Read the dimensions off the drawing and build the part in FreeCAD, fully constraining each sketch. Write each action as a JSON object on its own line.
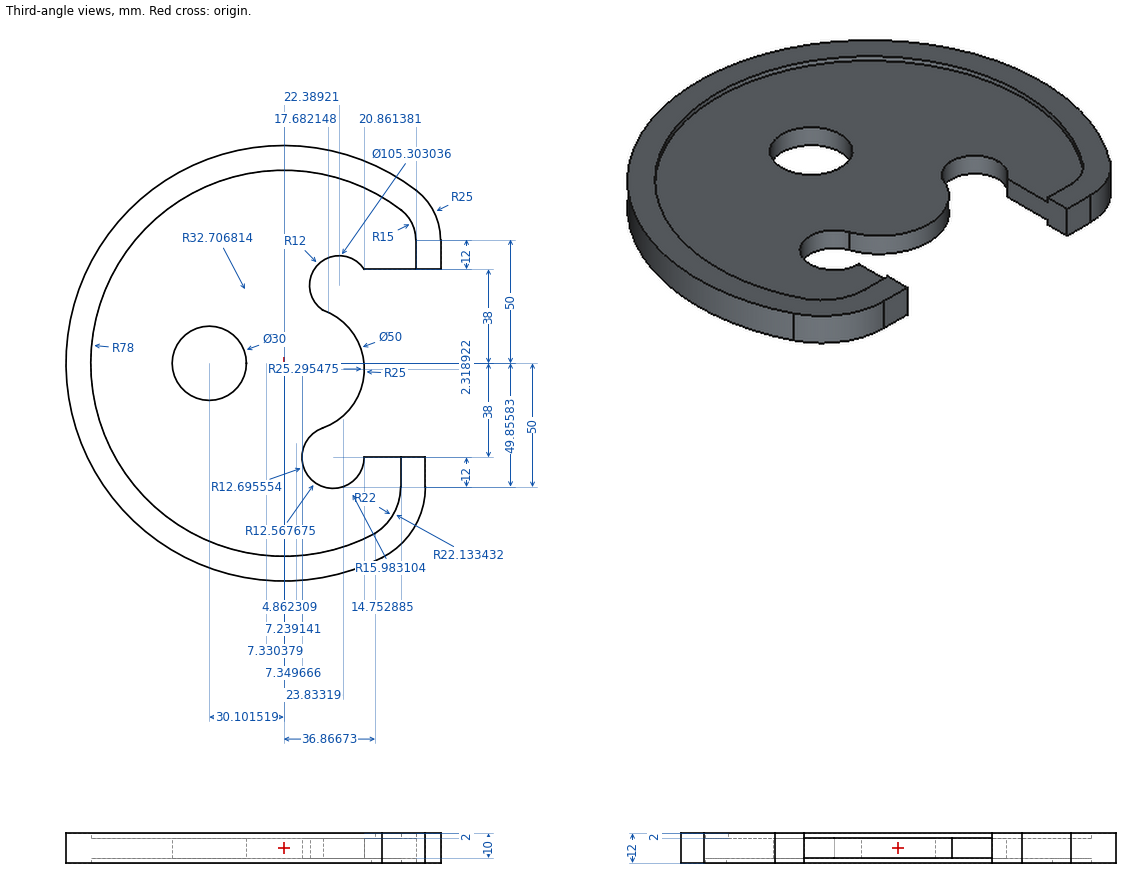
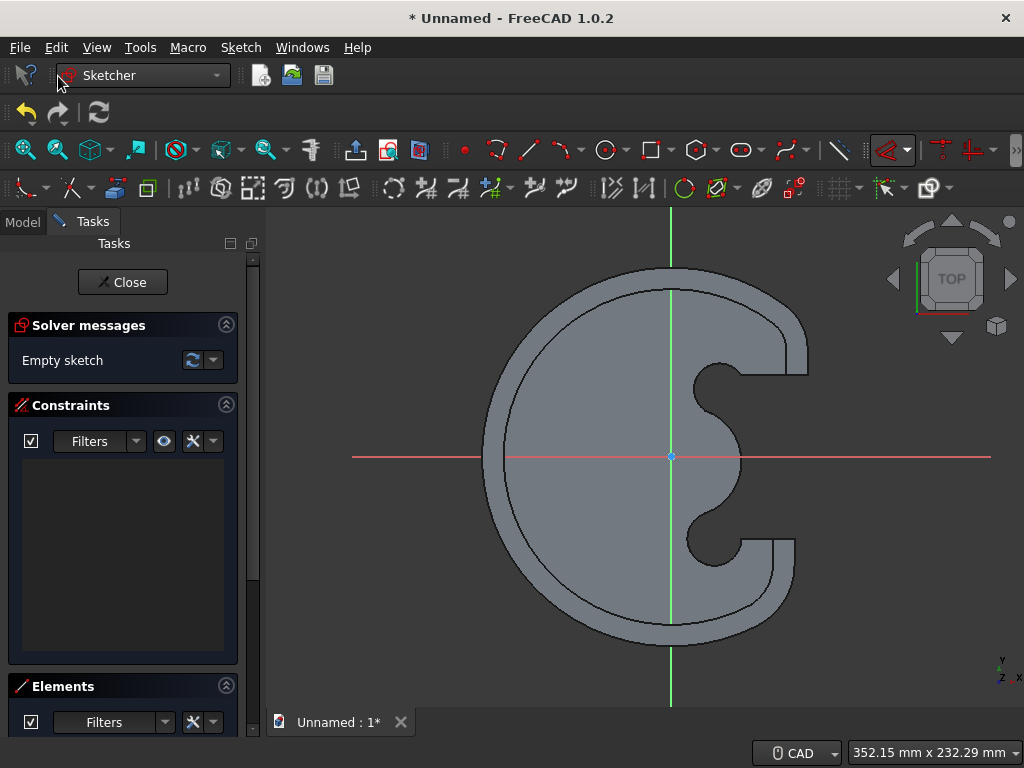
{"action": "scroll", "coordinate": [638, 457], "scroll_direction": "up", "scroll_amount": 7}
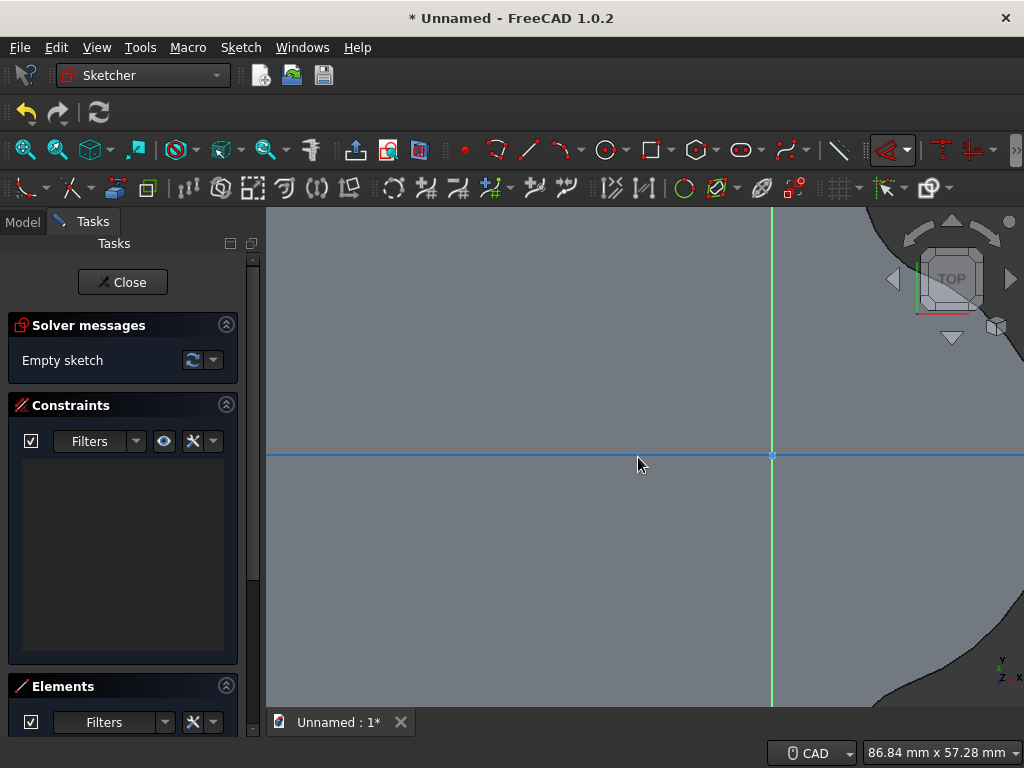
{"action": "key", "text": "g c"}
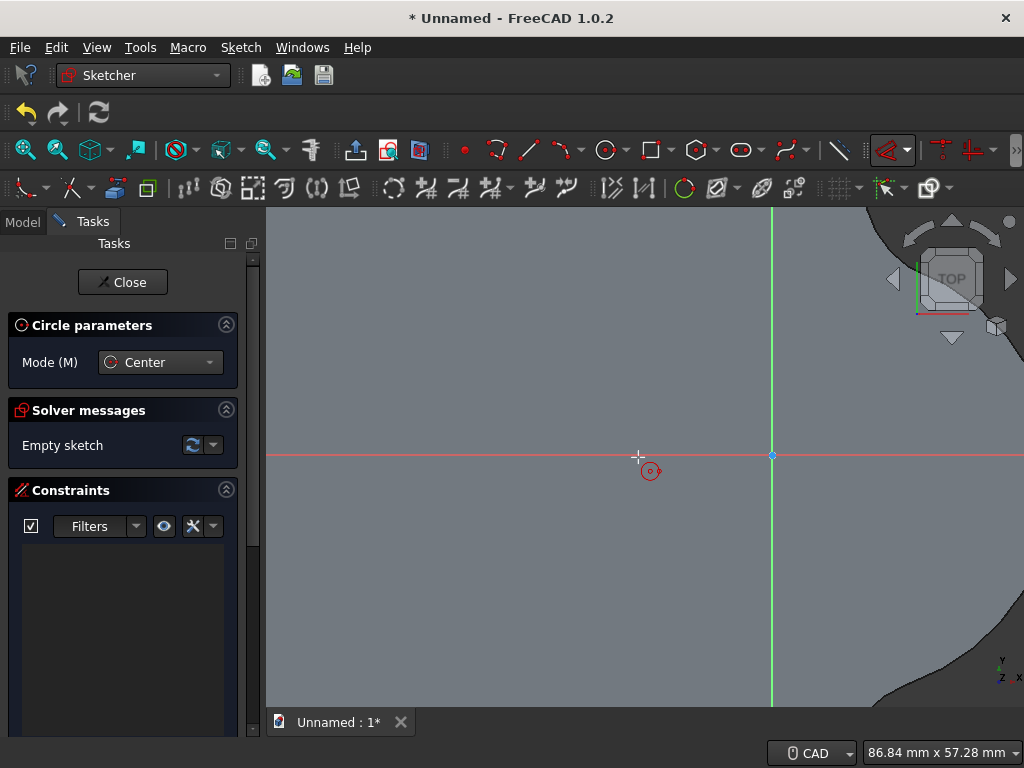
{"action": "left_click", "coordinate": [509, 455]}
{"action": "left_click", "coordinate": [602, 363]}
{"action": "key", "text": "Escape"}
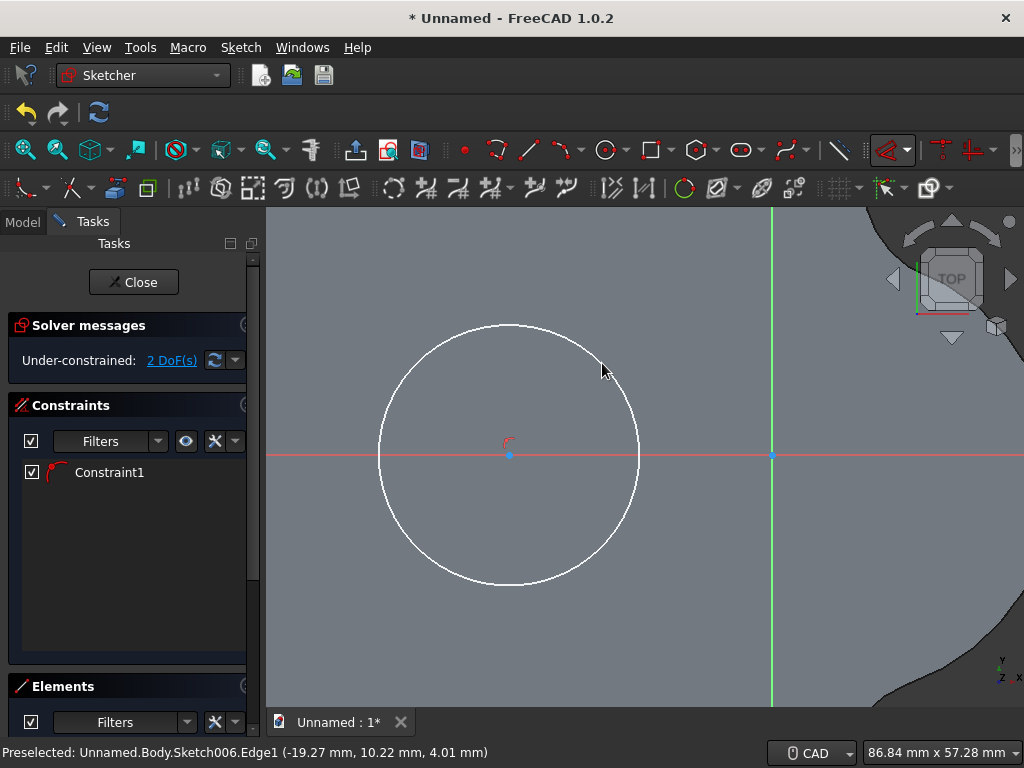
{"action": "left_click", "coordinate": [601, 363]}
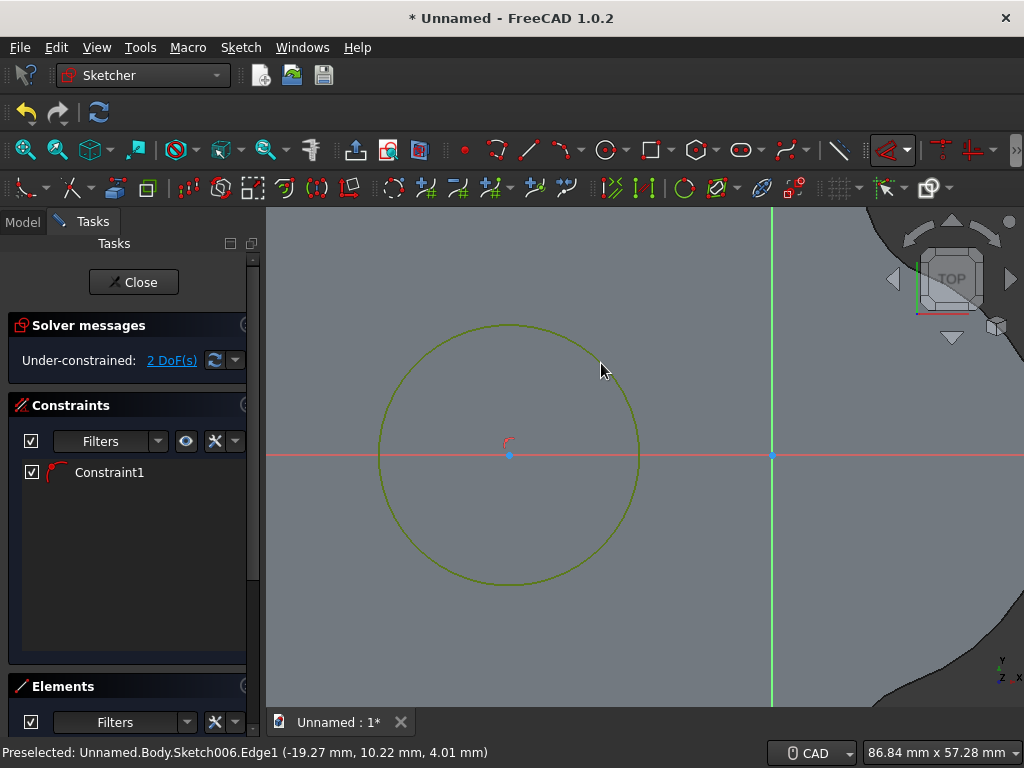
{"action": "key", "text": "k o"}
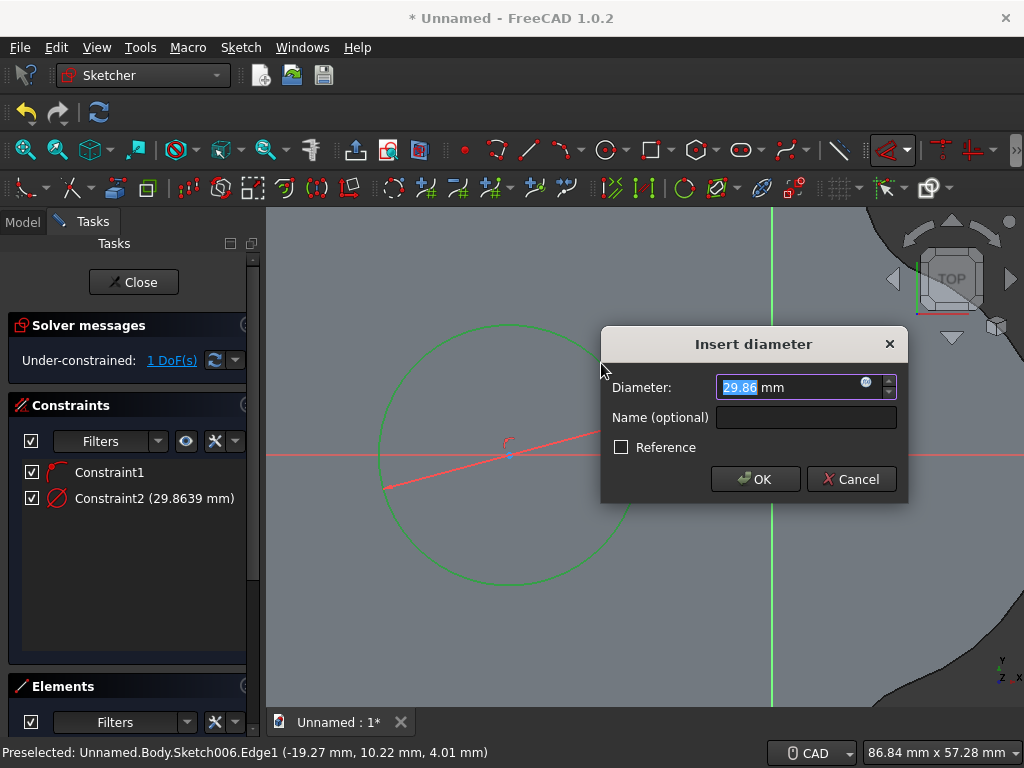
{"action": "type", "text": "30"}
{"action": "key", "text": "Return"}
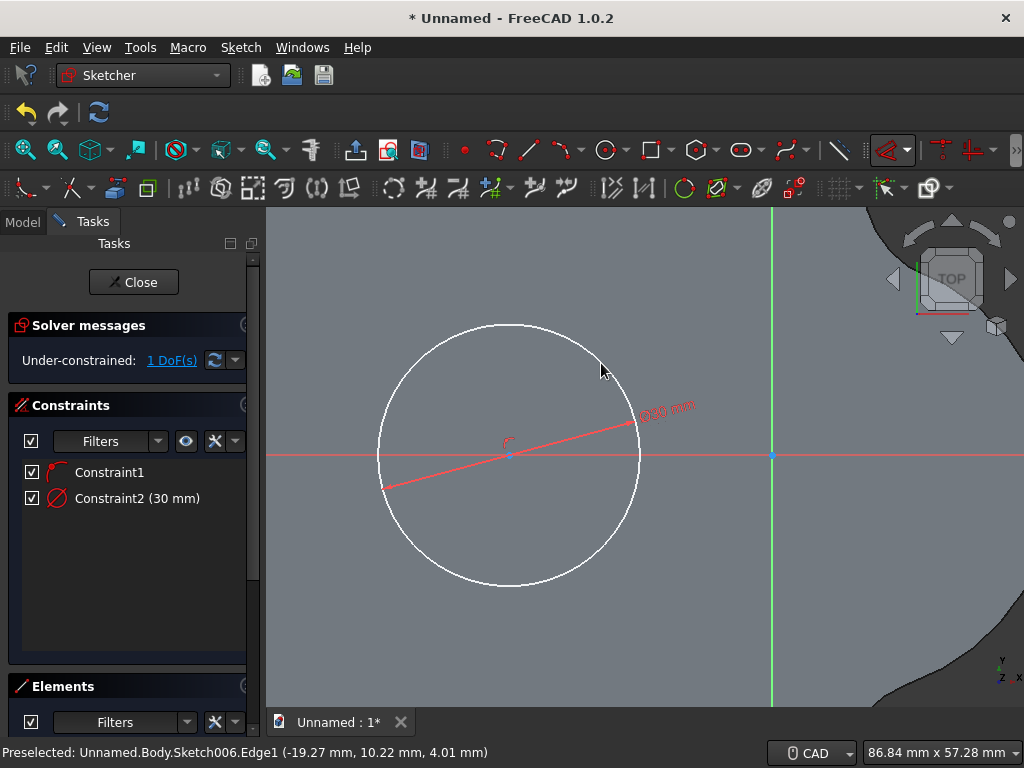
{"action": "left_click", "coordinate": [509, 455]}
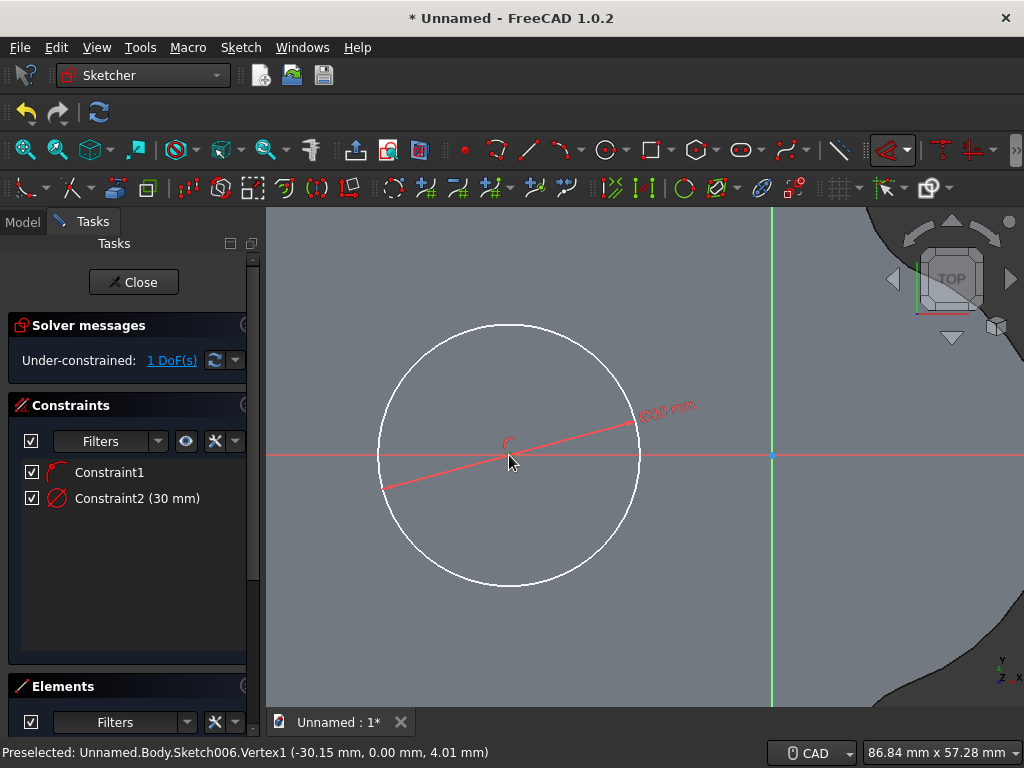
{"action": "key", "text": "l"}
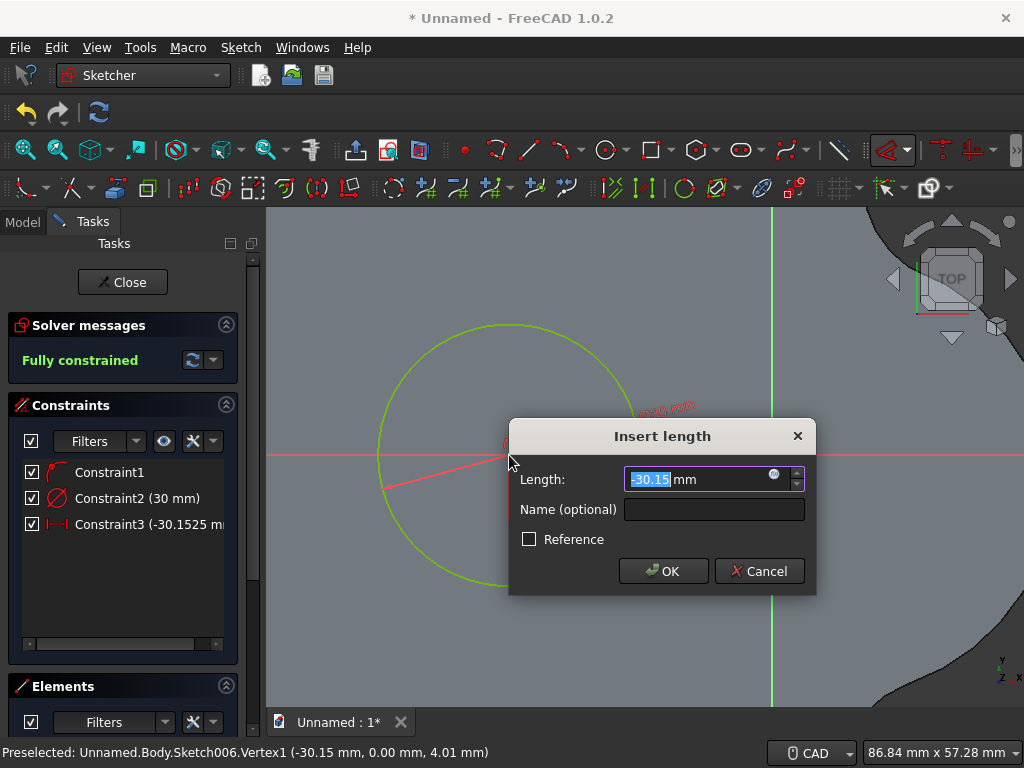
{"action": "type", "text": "-30.101519"}
{"action": "key", "text": "Return"}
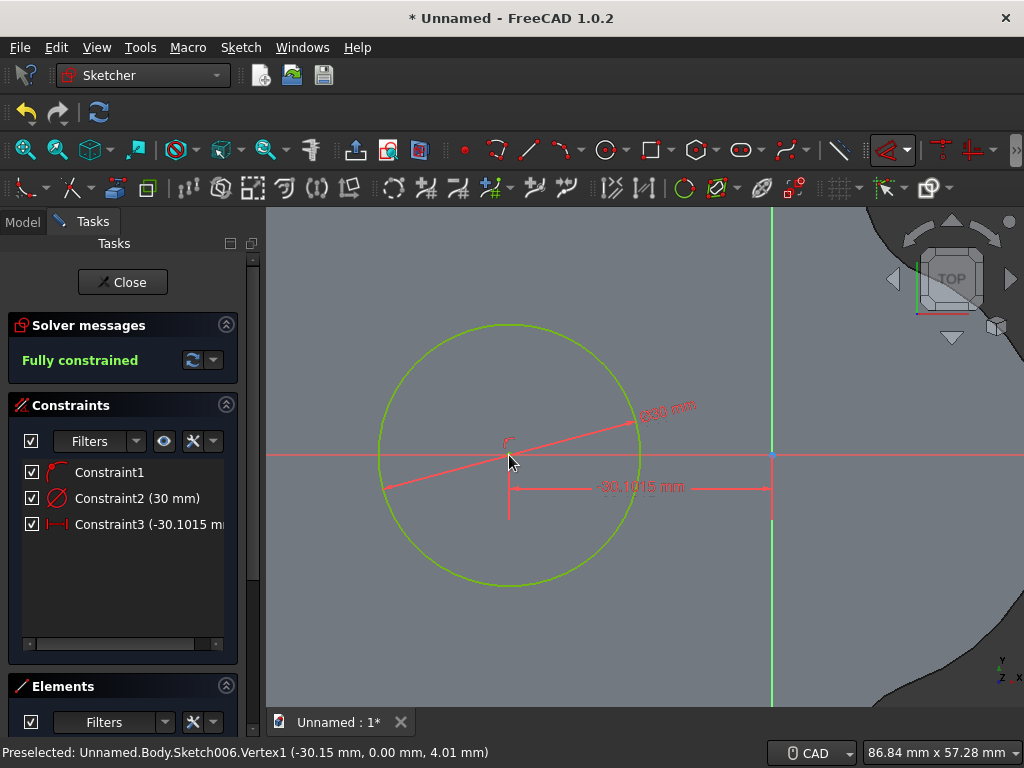
{"action": "left_click", "coordinate": [123, 282]}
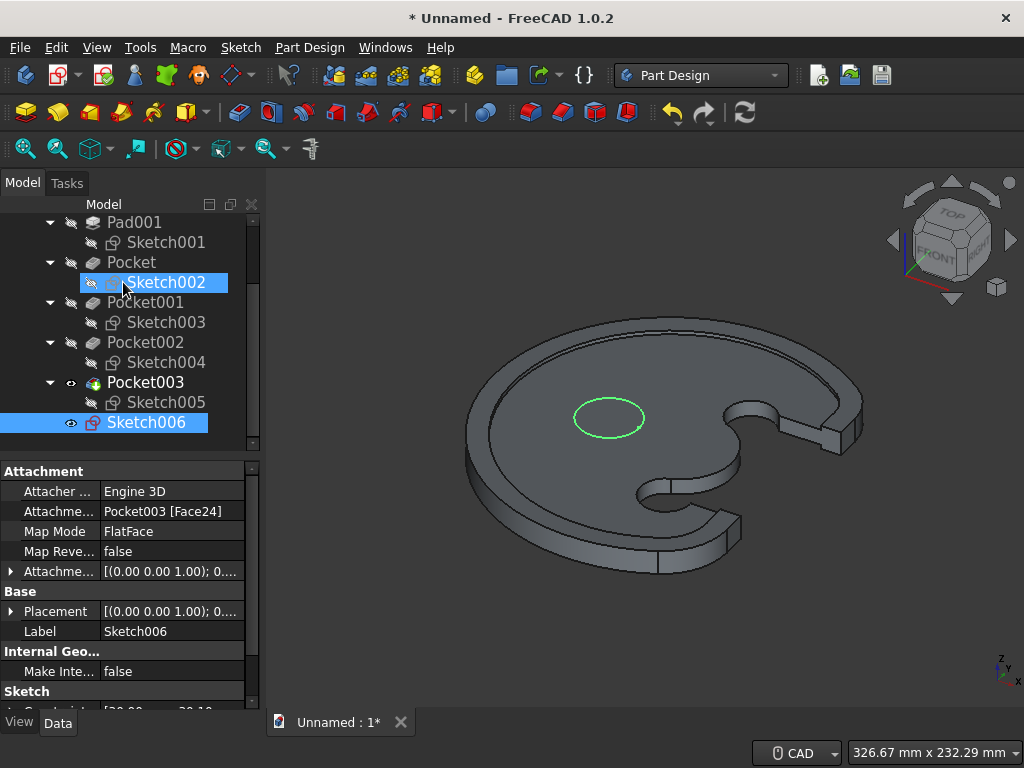
{"action": "left_click", "coordinate": [240, 112]}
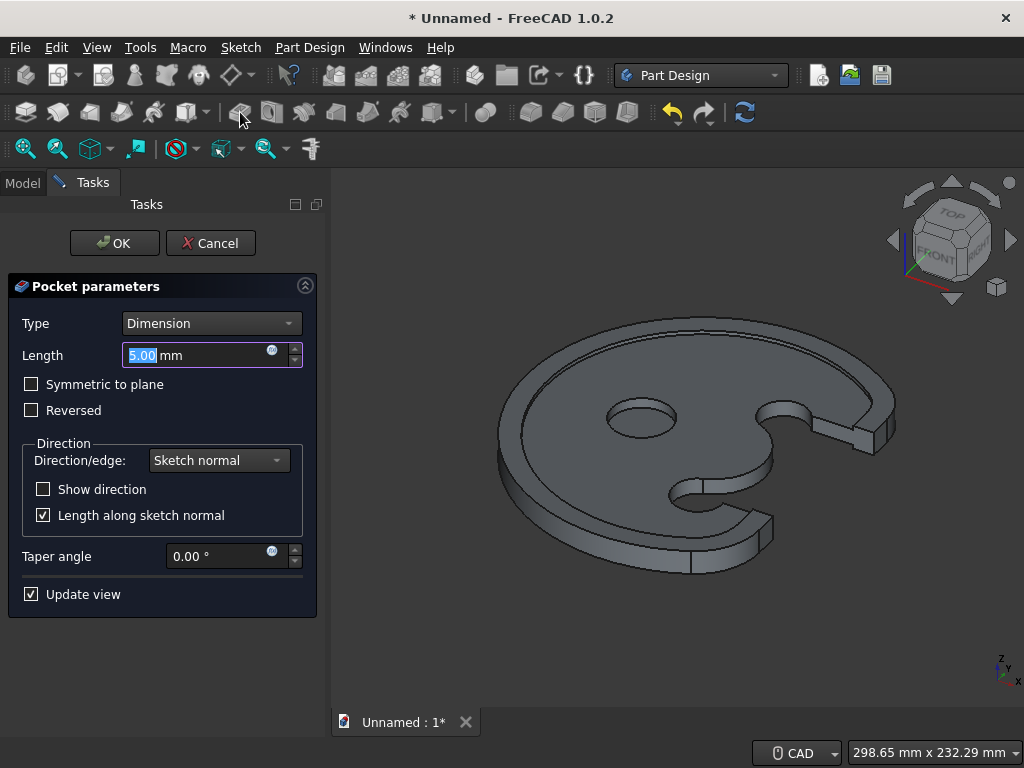
{"action": "left_click", "coordinate": [212, 324]}